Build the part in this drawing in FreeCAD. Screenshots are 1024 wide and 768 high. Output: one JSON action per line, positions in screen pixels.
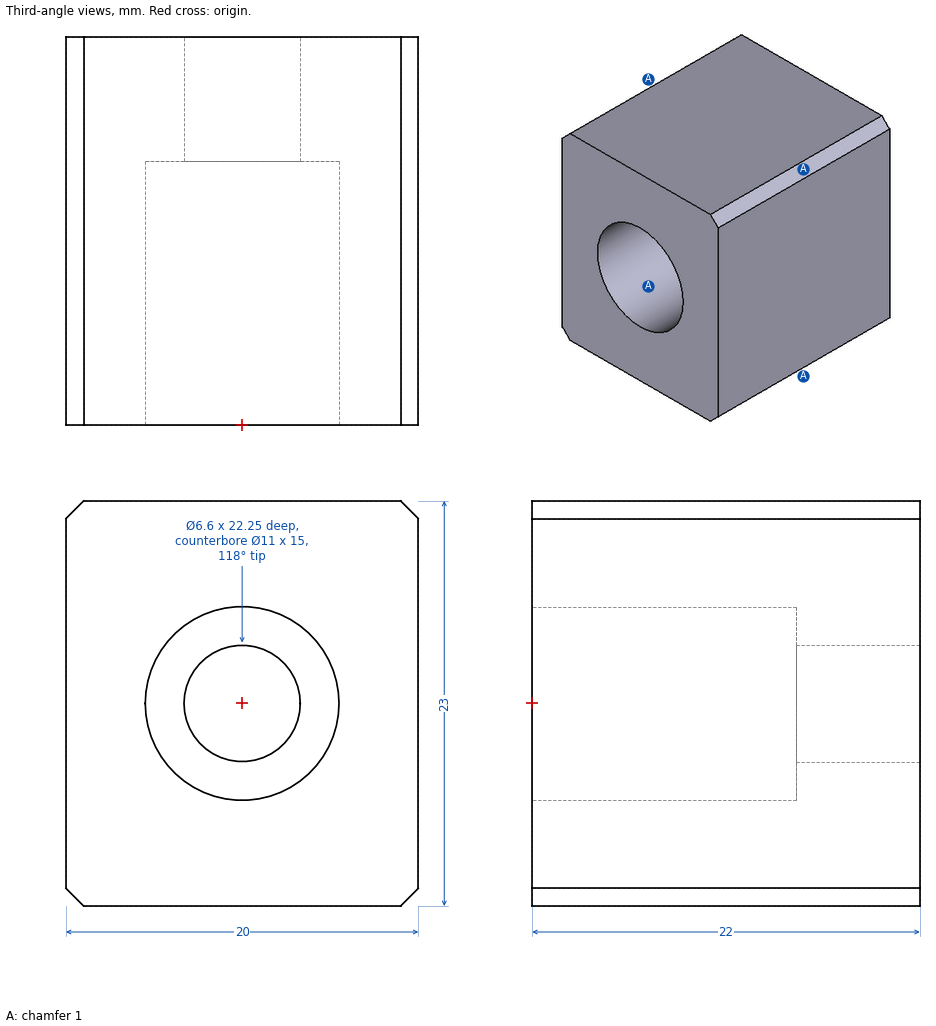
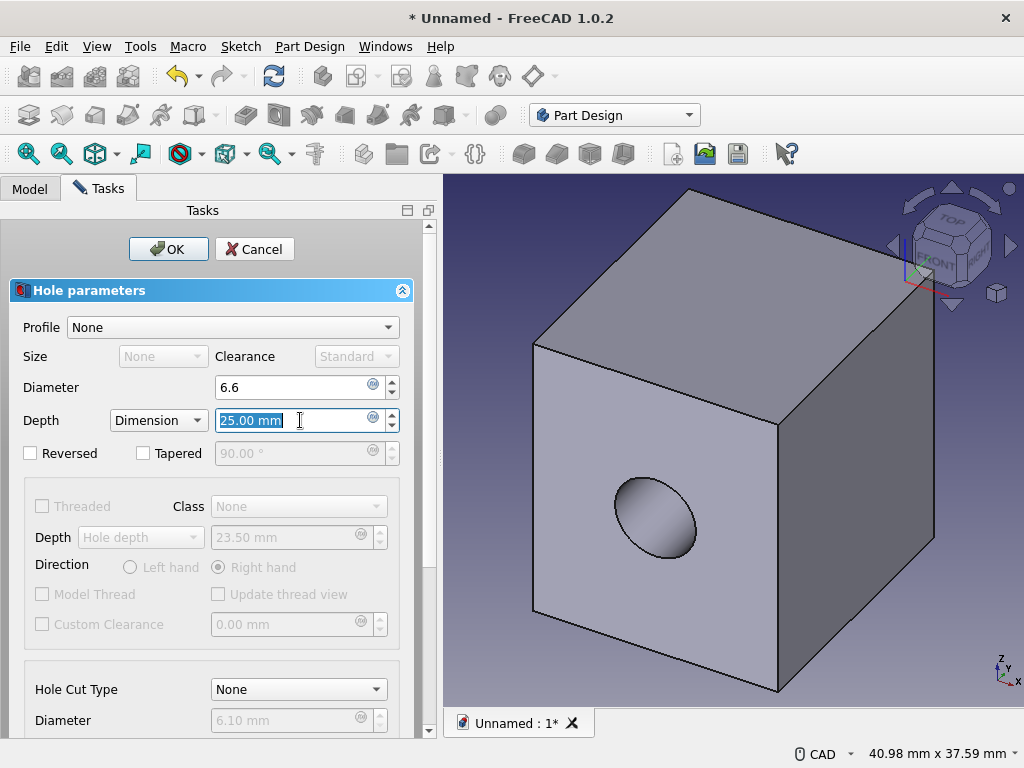
{"action": "type", "text": "22.25"}
{"action": "key", "text": "Tab"}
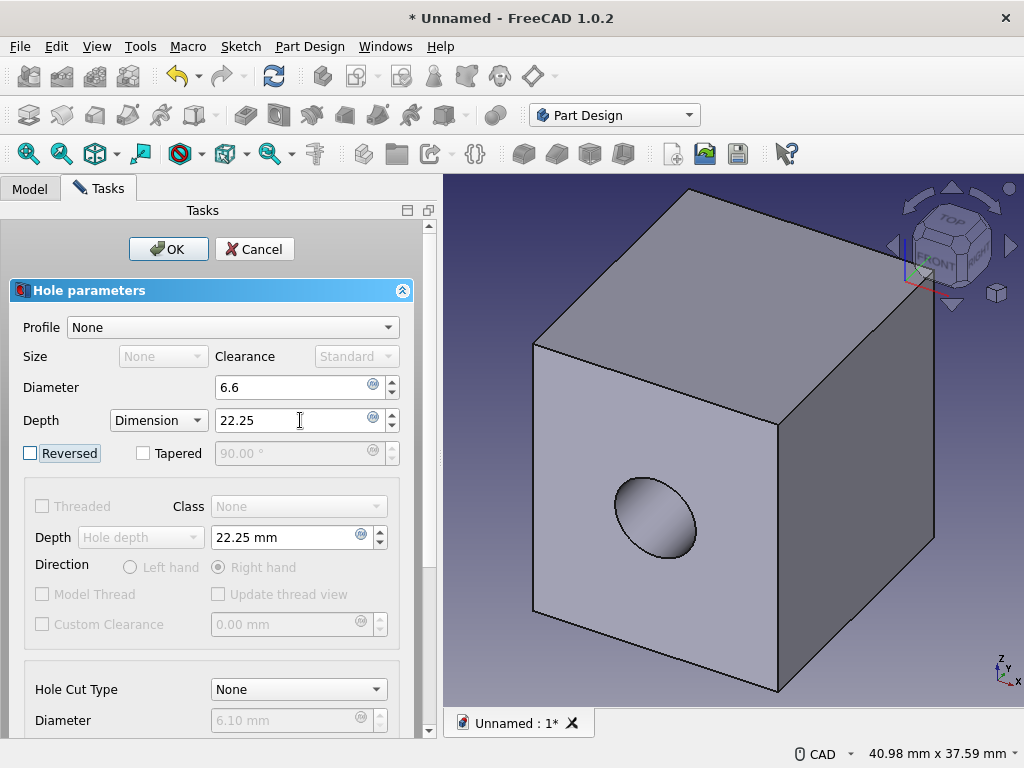
{"action": "left_click", "coordinate": [300, 690]}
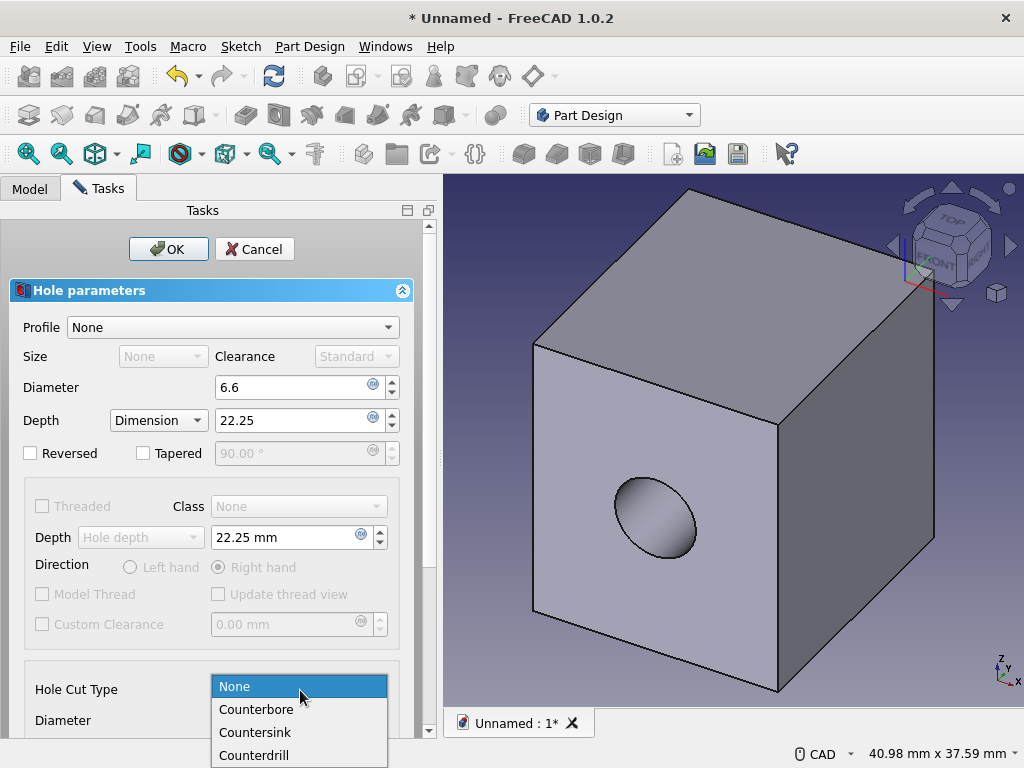
{"action": "left_click", "coordinate": [298, 710]}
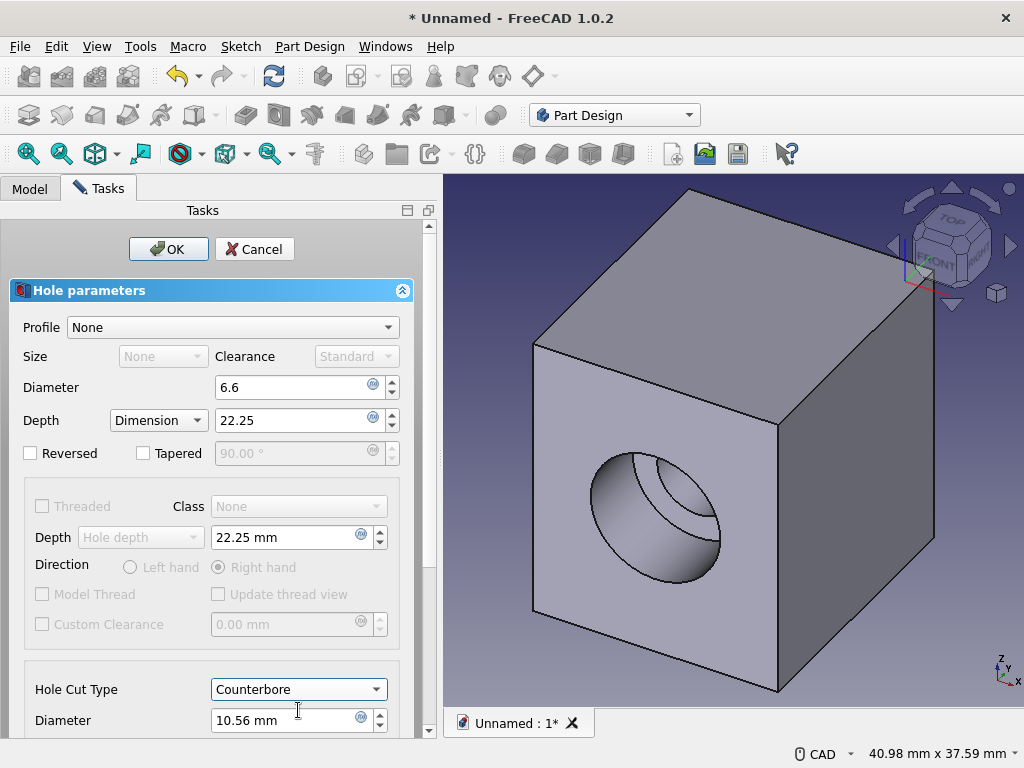
{"action": "triple_click", "coordinate": [292, 720]}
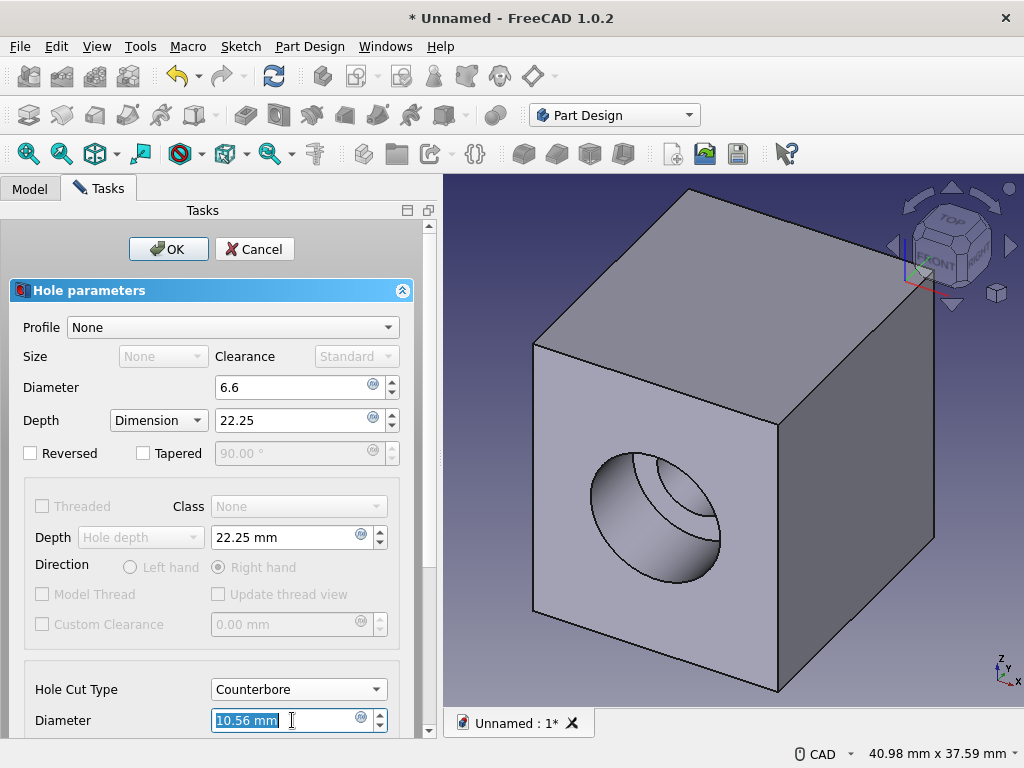
{"action": "type", "text": "11"}
{"action": "key", "text": "Tab"}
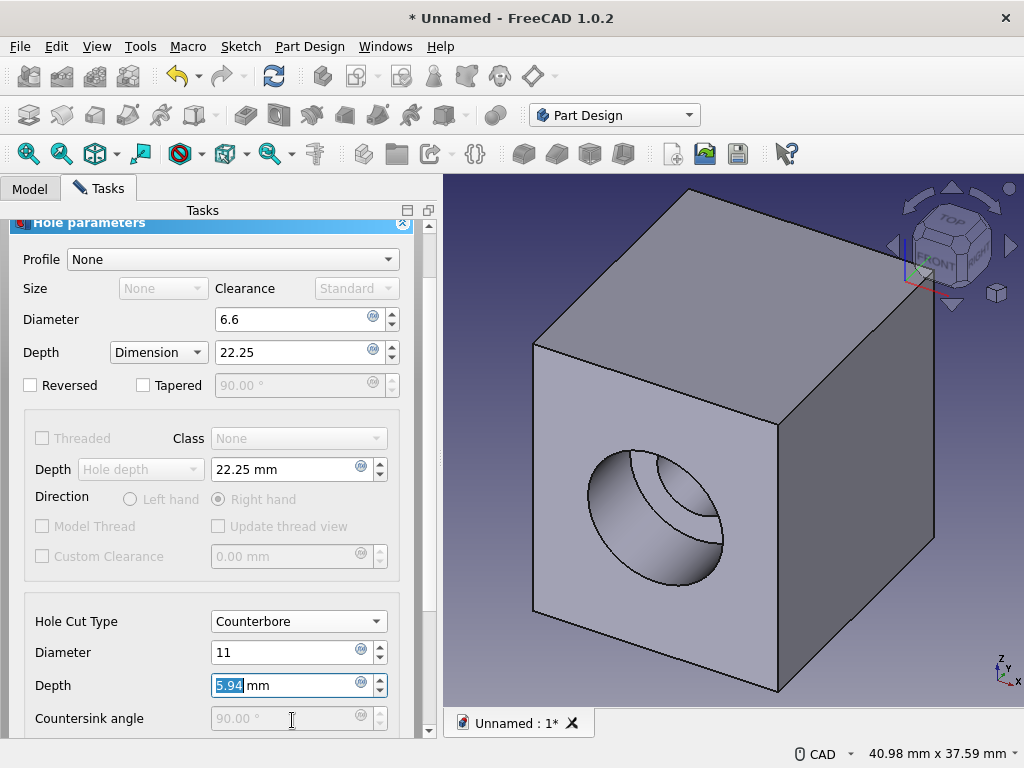
{"action": "type", "text": "15"}
{"action": "key", "text": "Tab"}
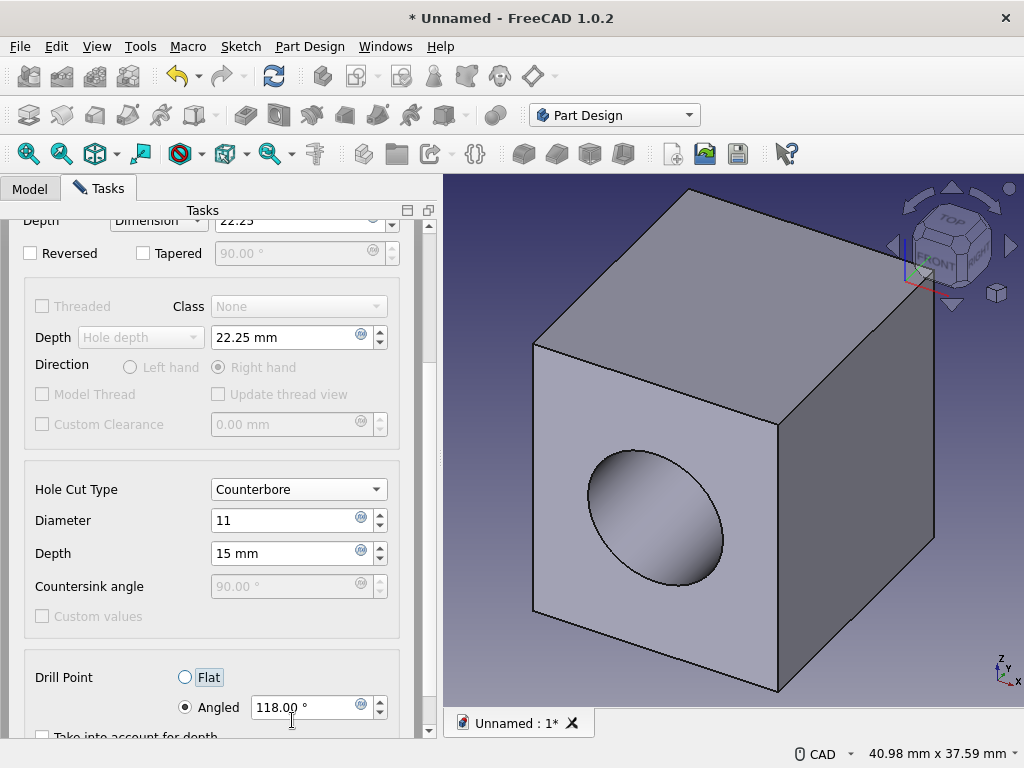
{"action": "scroll", "coordinate": [429, 479], "scroll_direction": "up", "scroll_amount": 5}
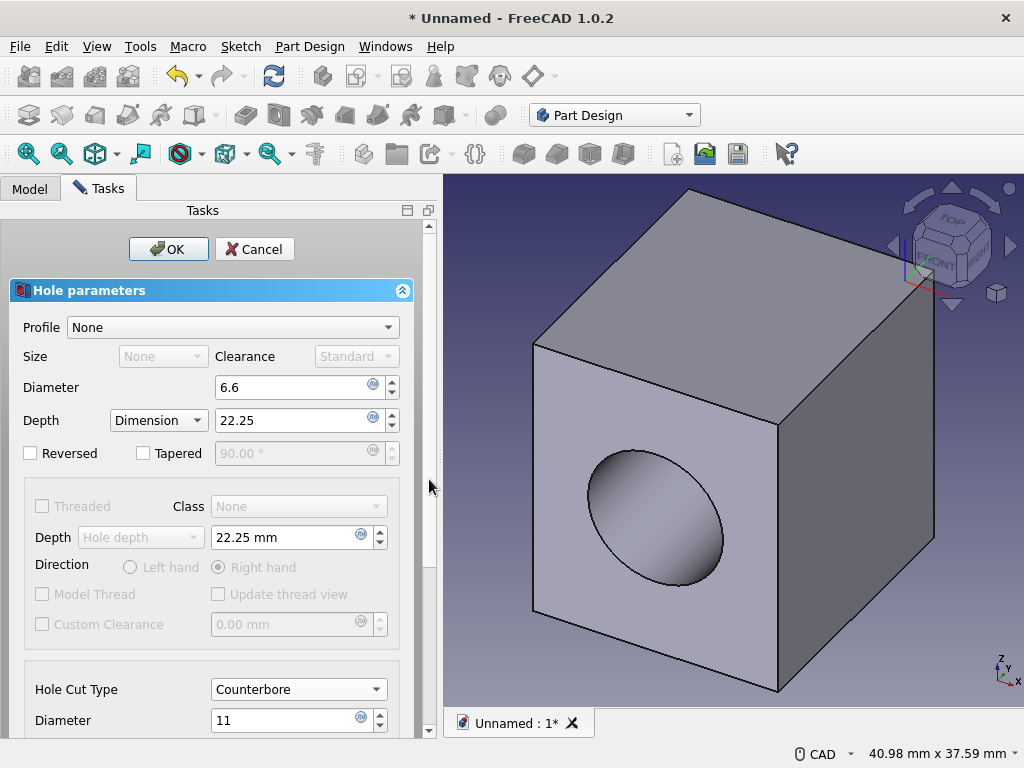
{"action": "left_click", "coordinate": [169, 249]}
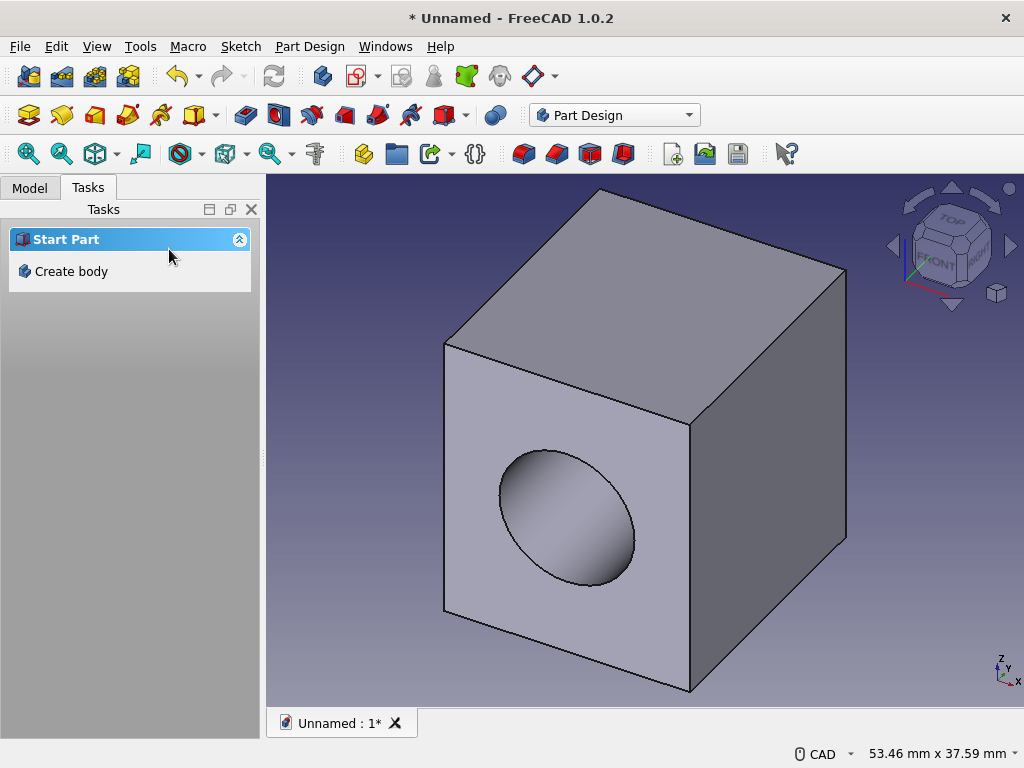
{"action": "left_click", "coordinate": [768, 347]}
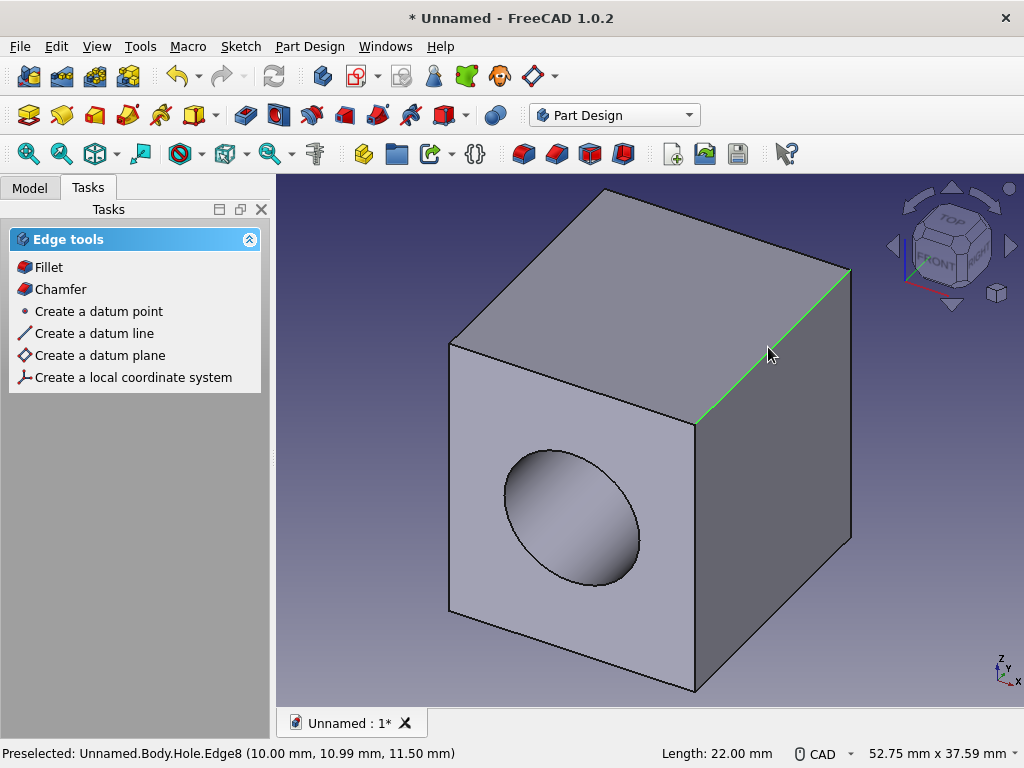
{"action": "key", "text": "0"}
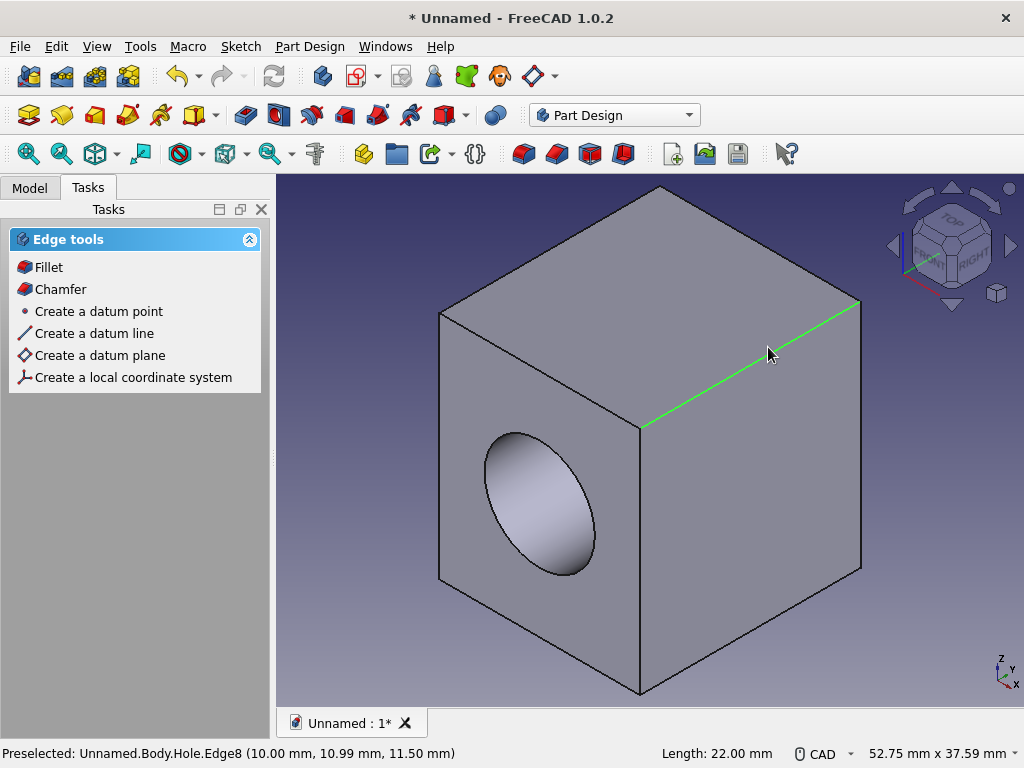
{"action": "key", "text": "2"}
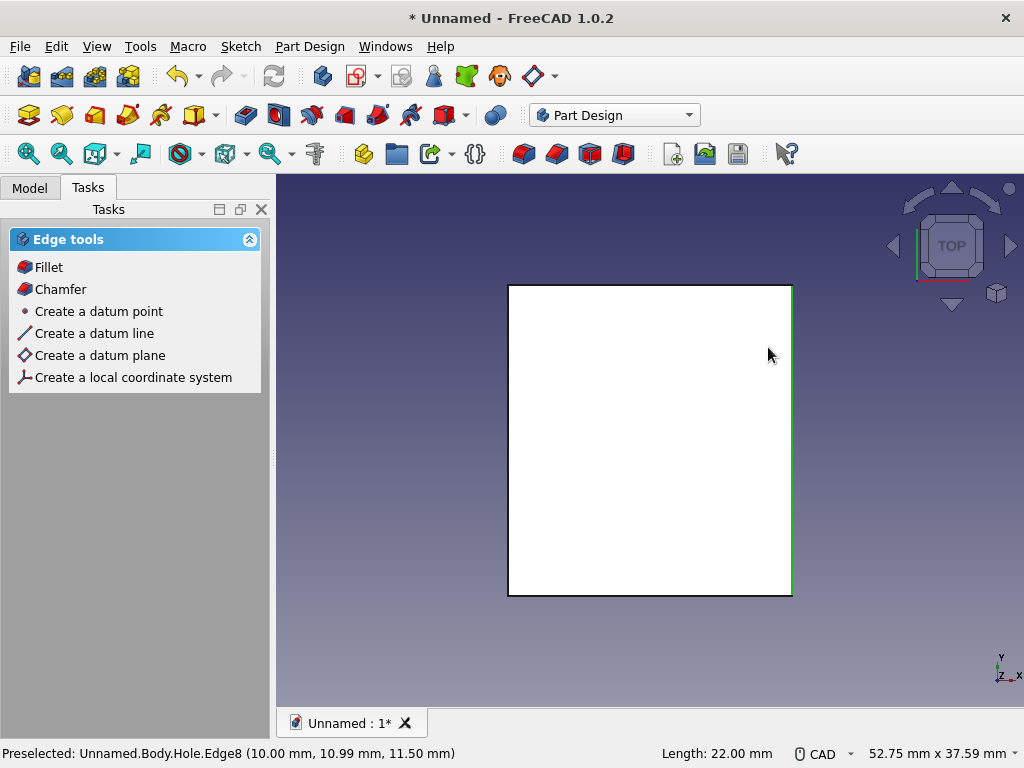
{"action": "left_click", "coordinate": [508, 440], "text": "ctrl"}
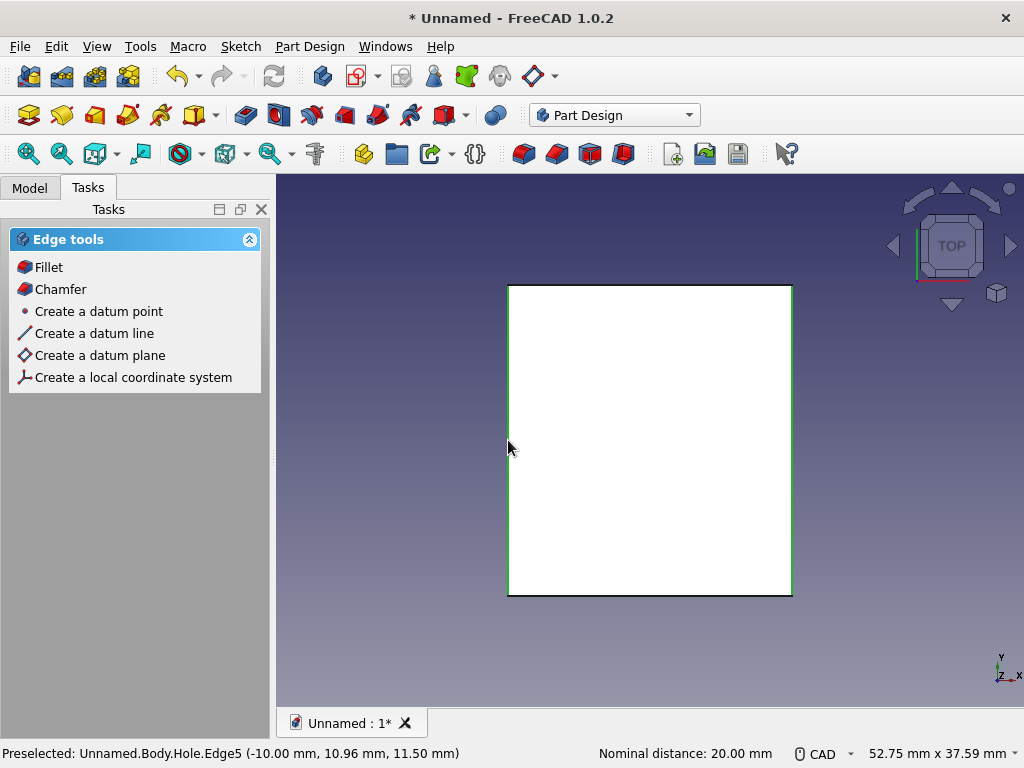
{"action": "key", "text": "1"}